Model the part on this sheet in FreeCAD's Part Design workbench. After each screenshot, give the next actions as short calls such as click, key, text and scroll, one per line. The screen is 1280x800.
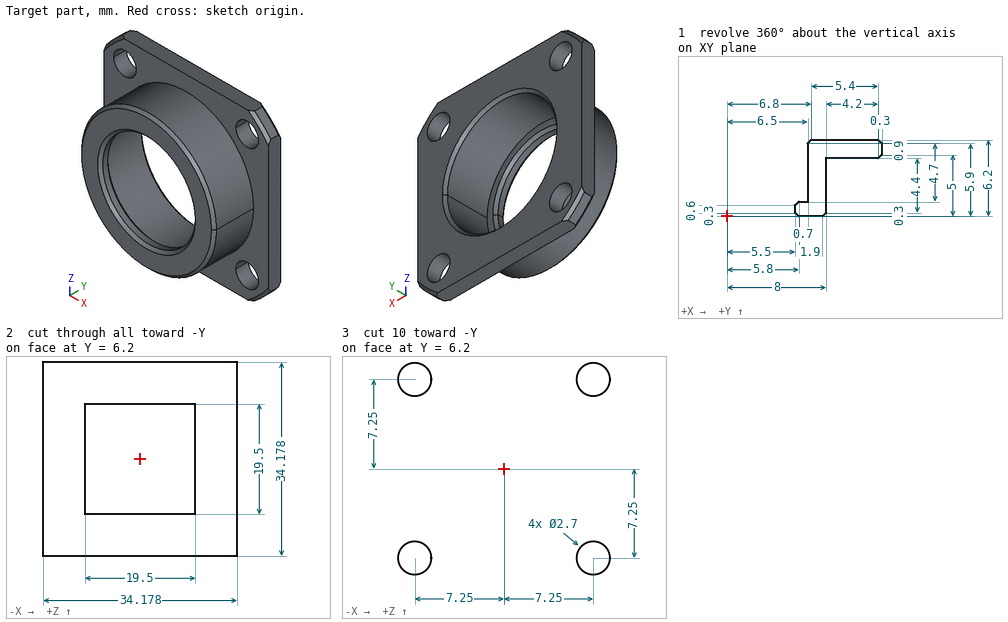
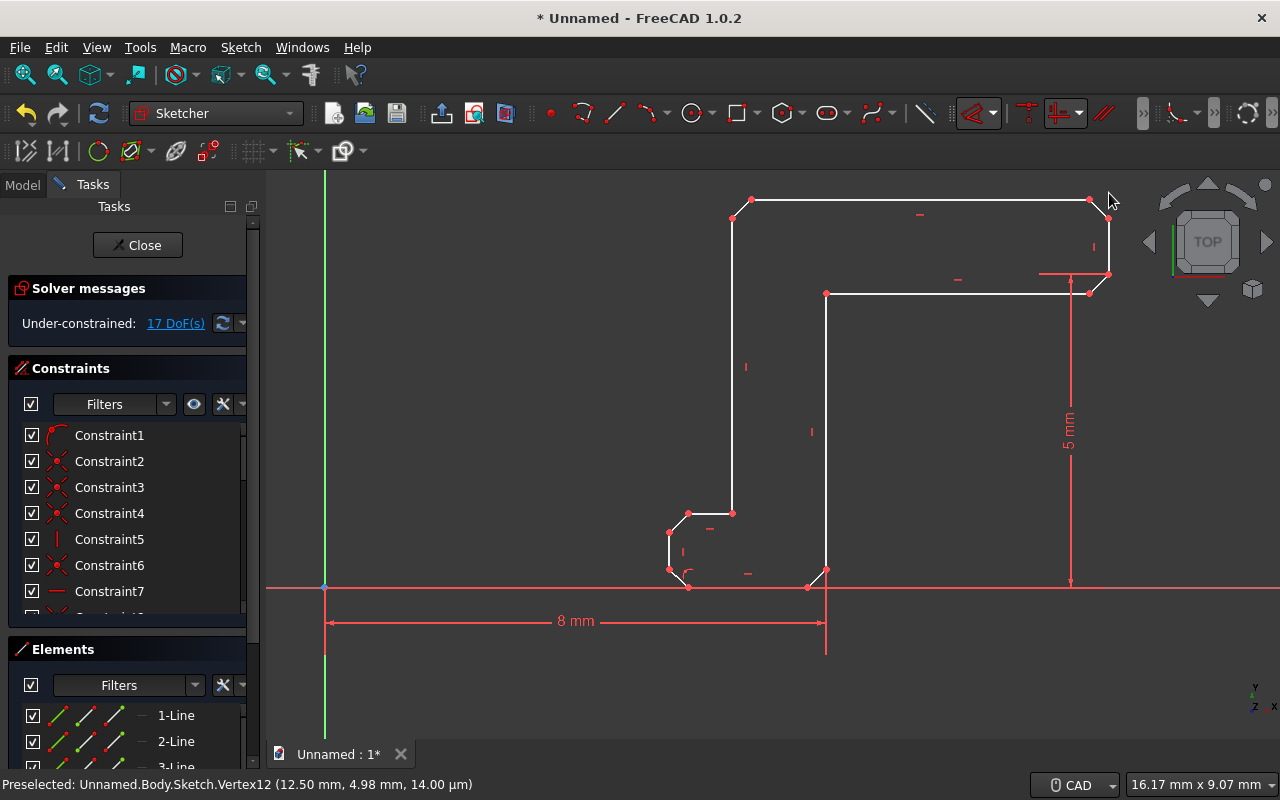
click(724, 588)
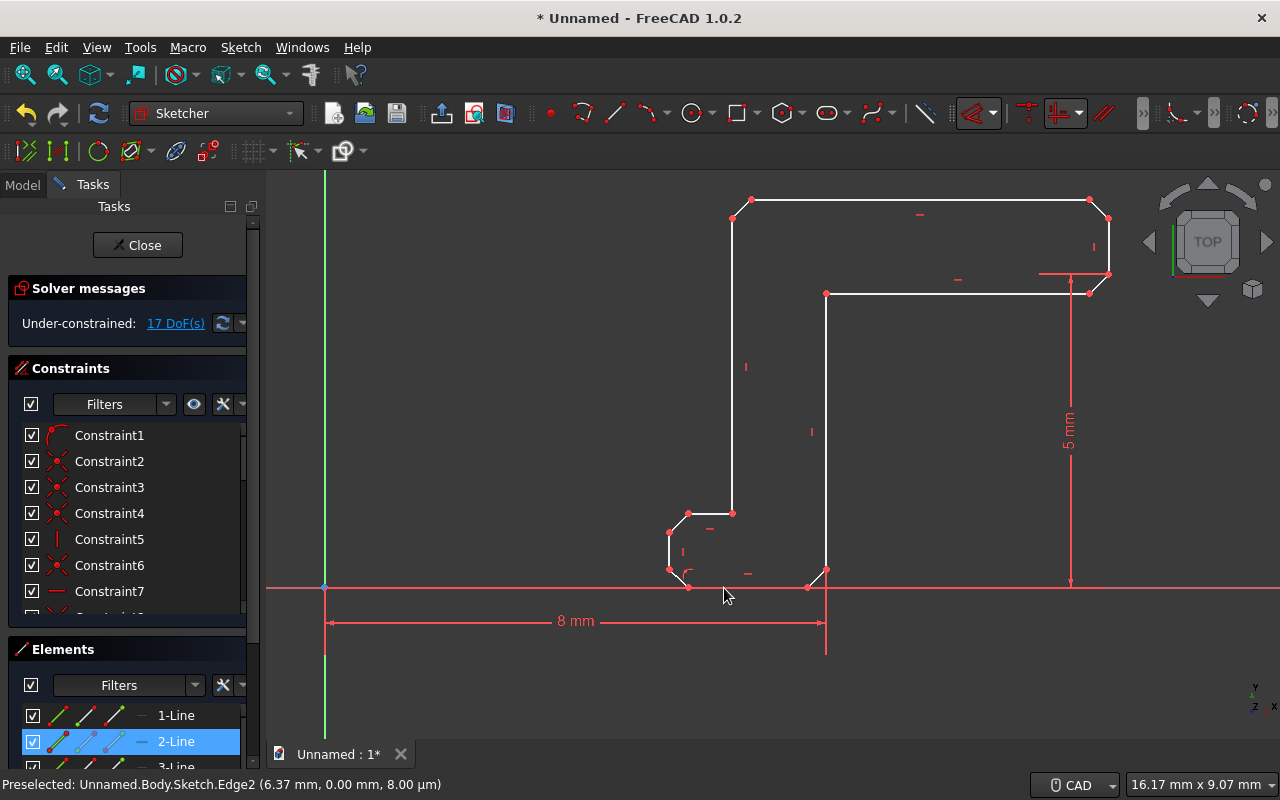
click(996, 114)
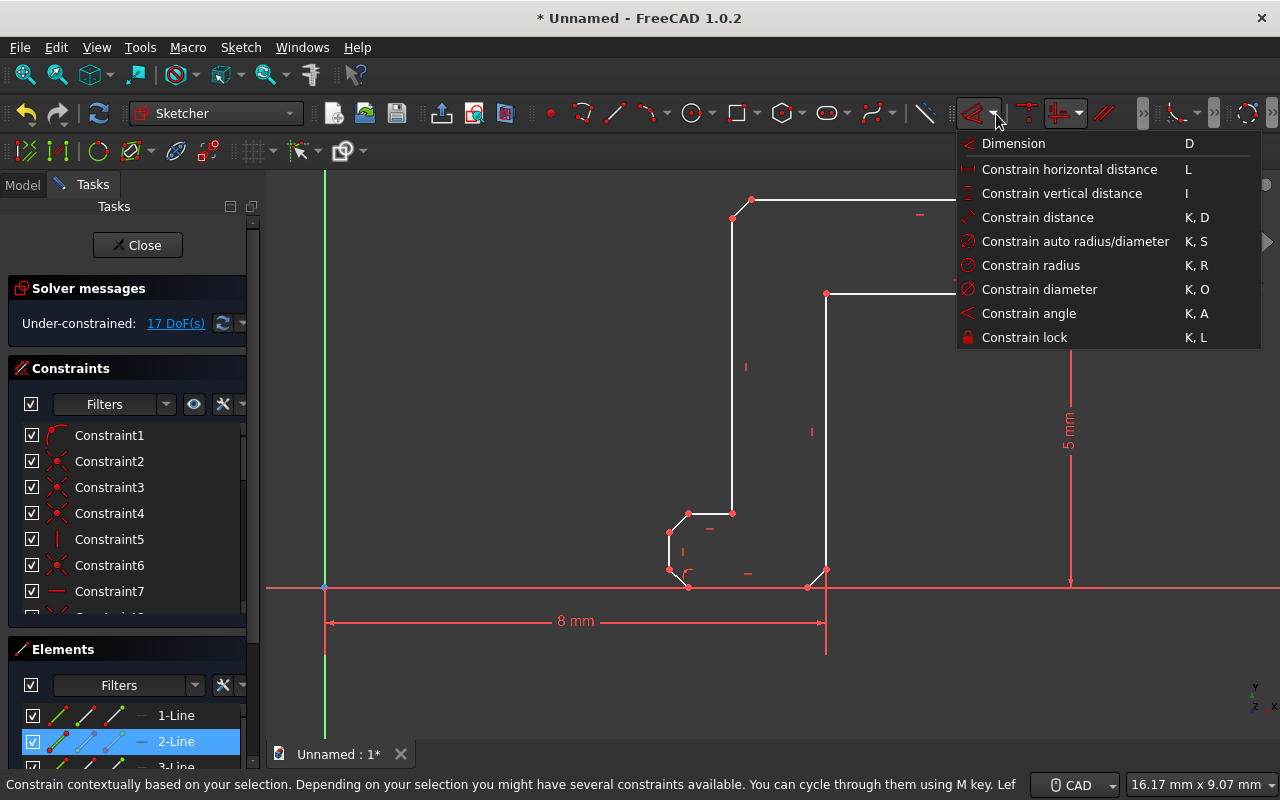
click(1109, 169)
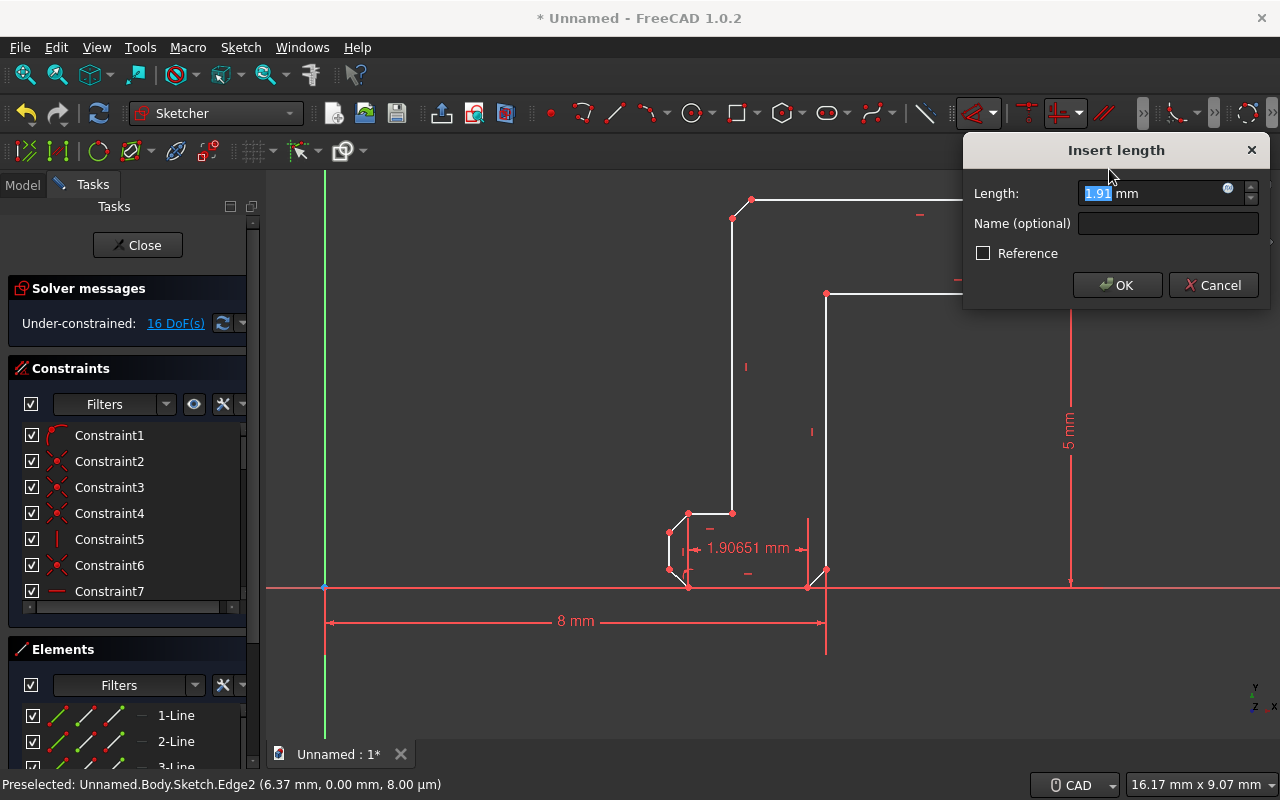
text(1.9)
key(Return)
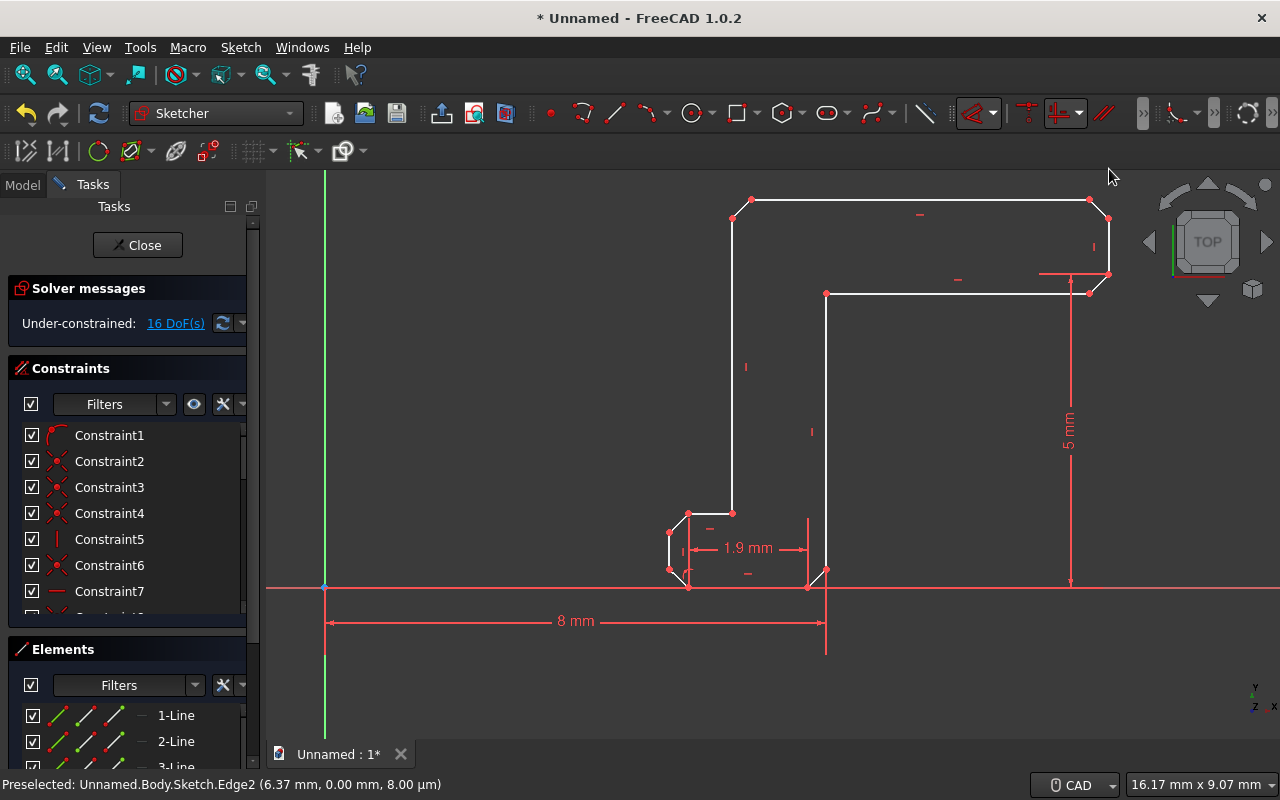
click(826, 487)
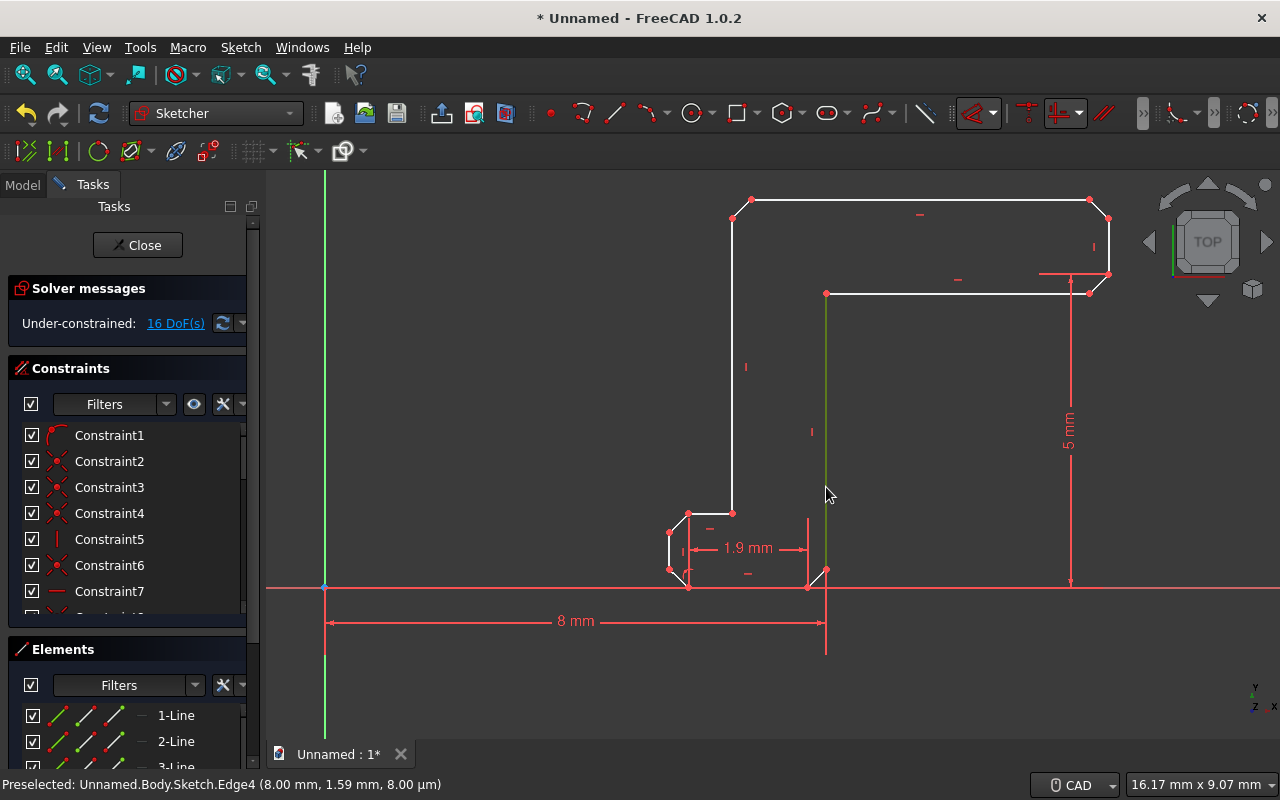
key(i)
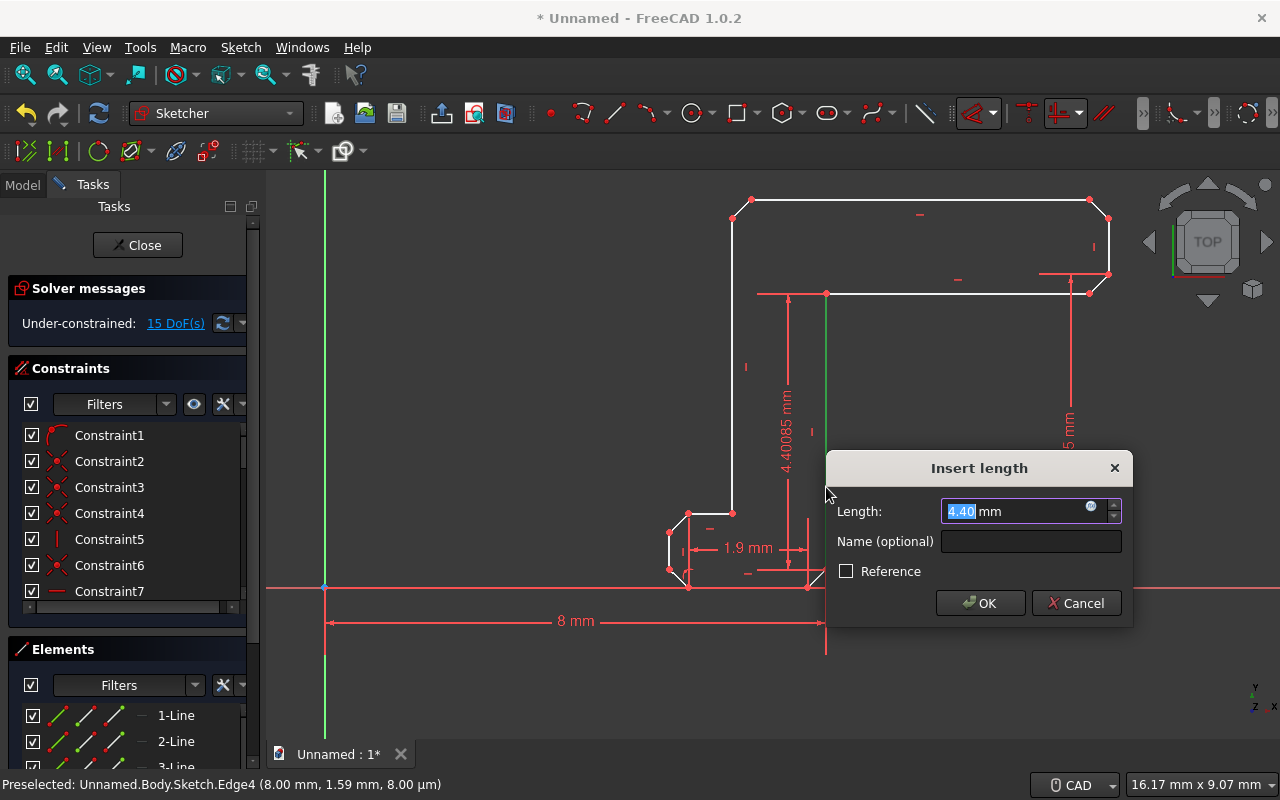
text(4.4)
key(Return)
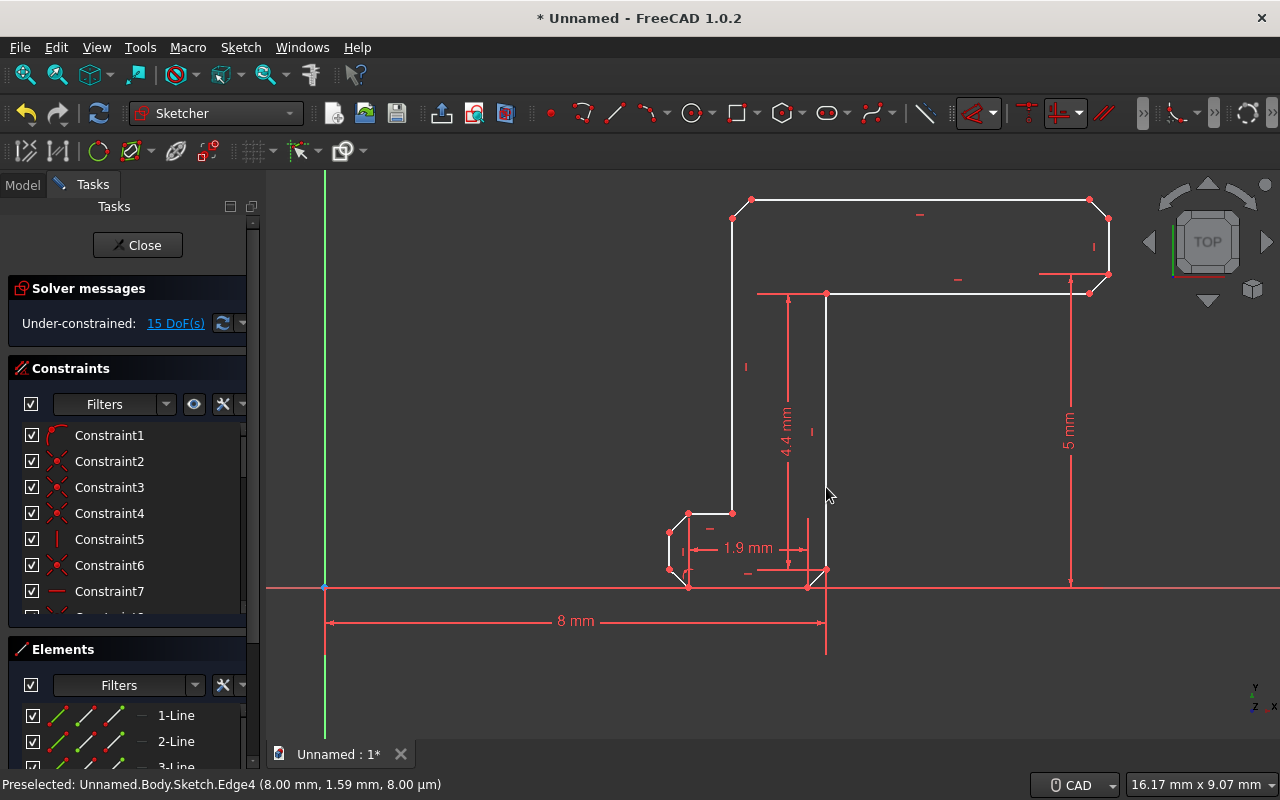
click(905, 294)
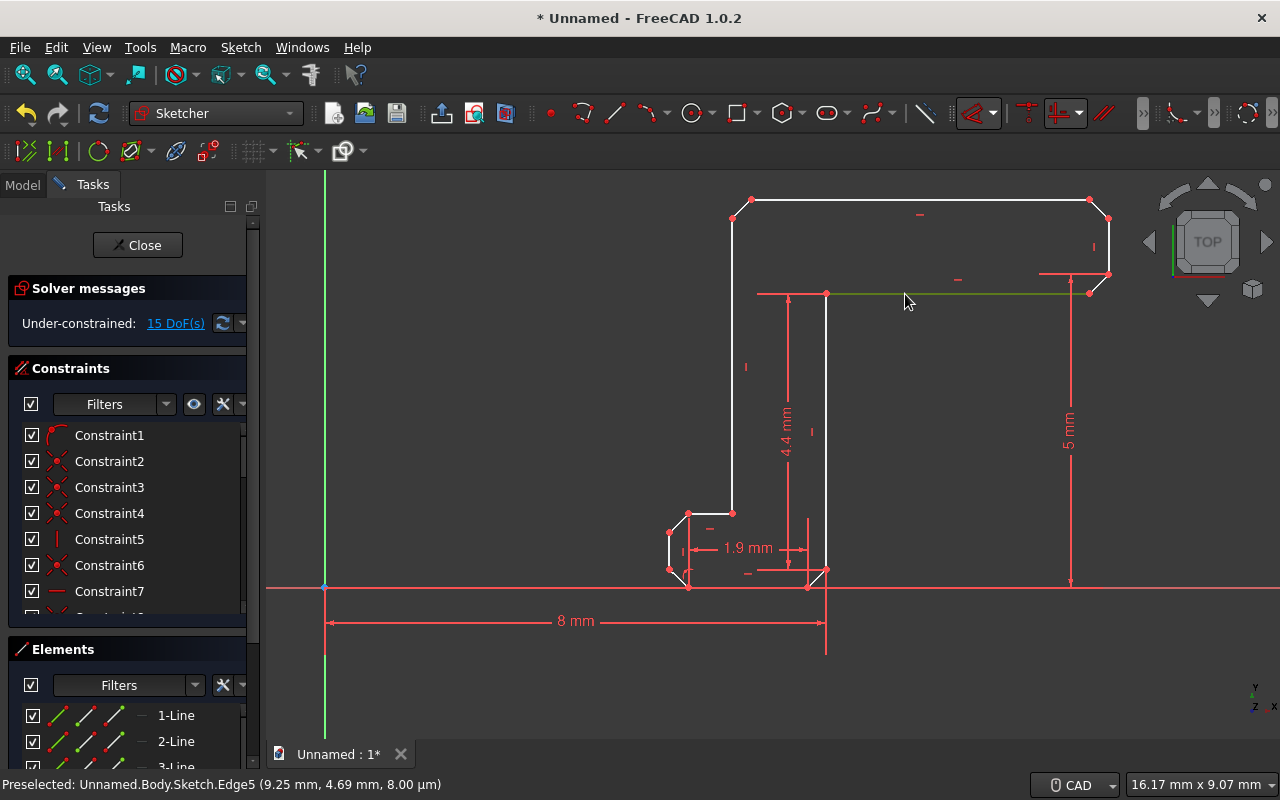
click(996, 114)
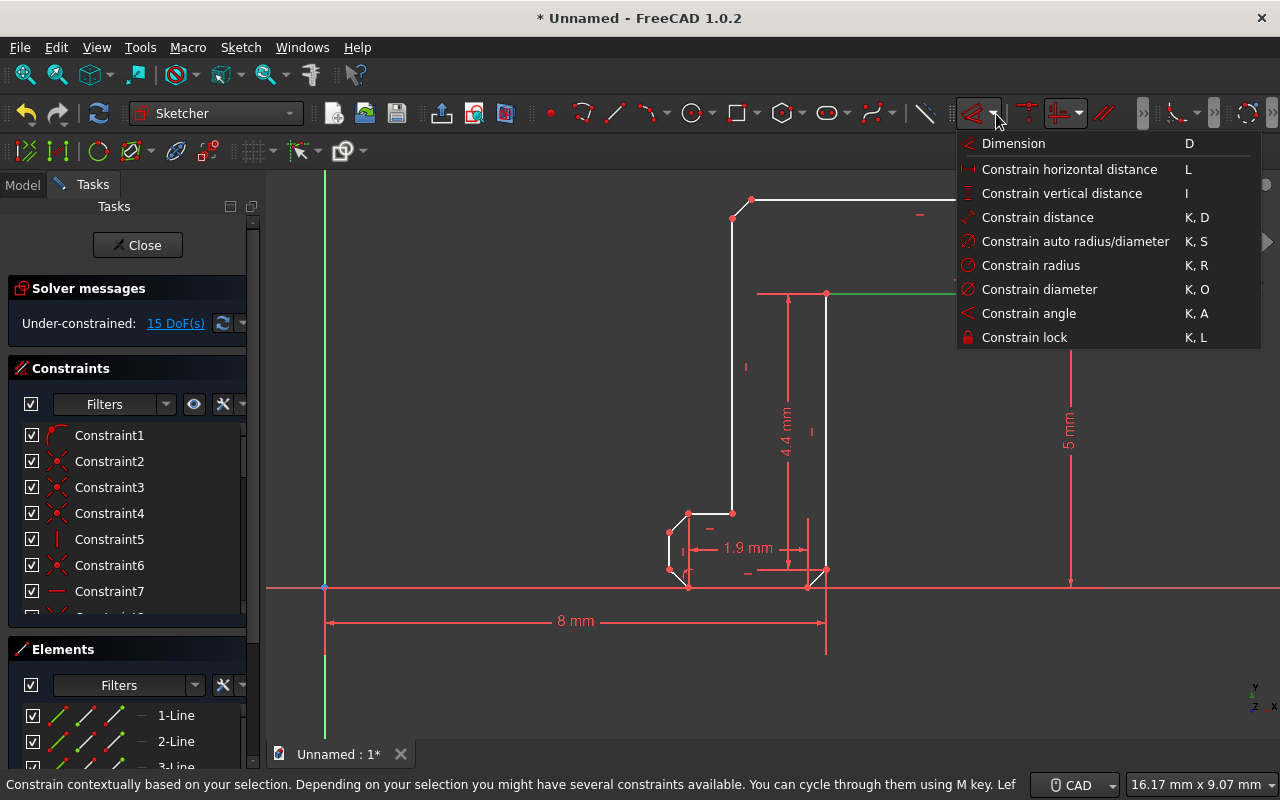
click(1109, 169)